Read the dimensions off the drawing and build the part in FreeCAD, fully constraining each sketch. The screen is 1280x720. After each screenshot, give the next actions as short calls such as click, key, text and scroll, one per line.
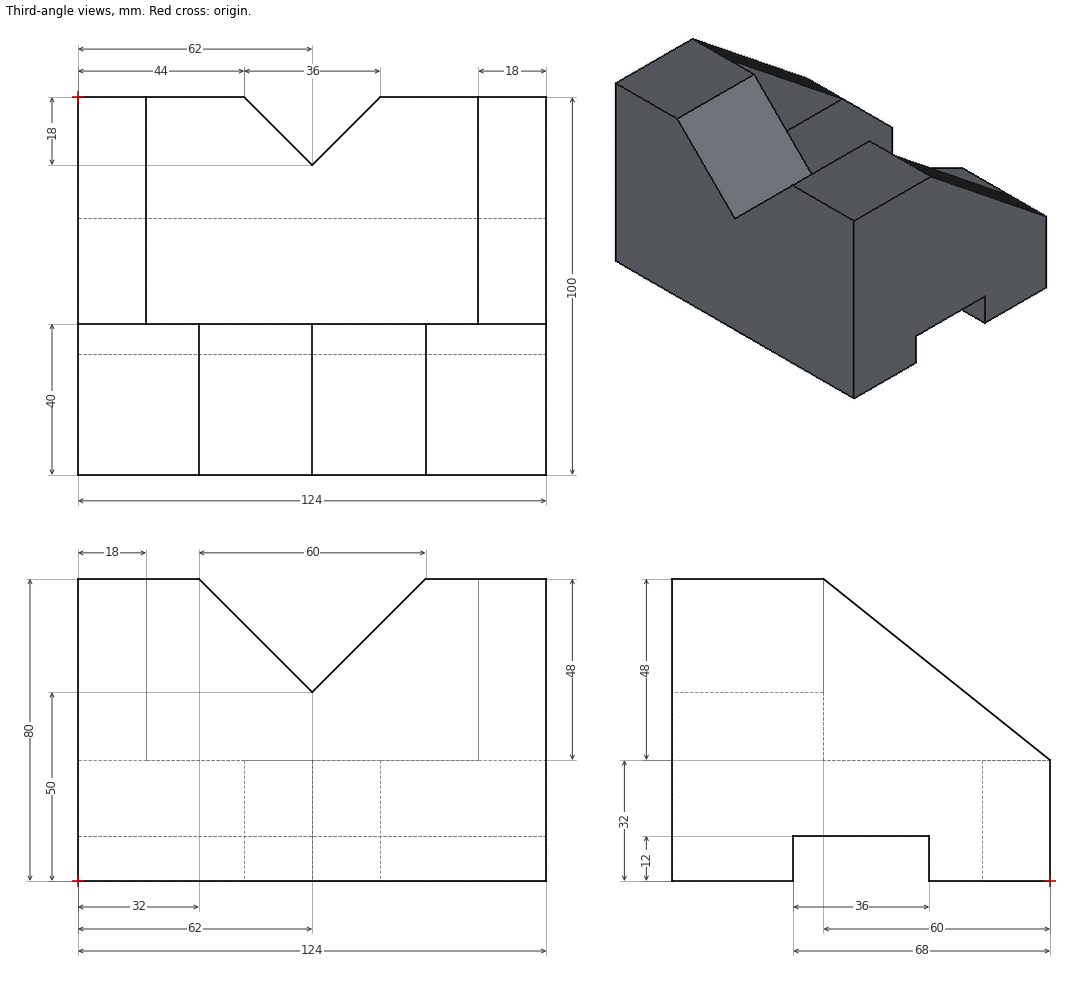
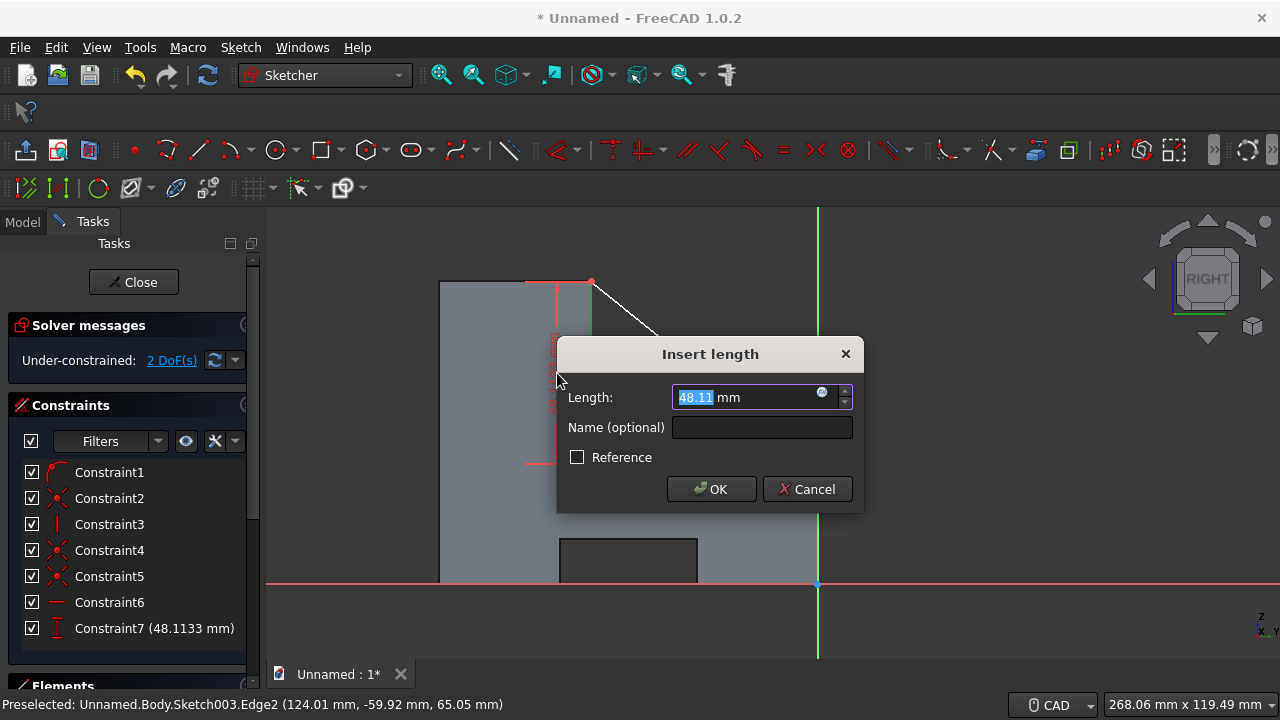
text(48)
key(Return)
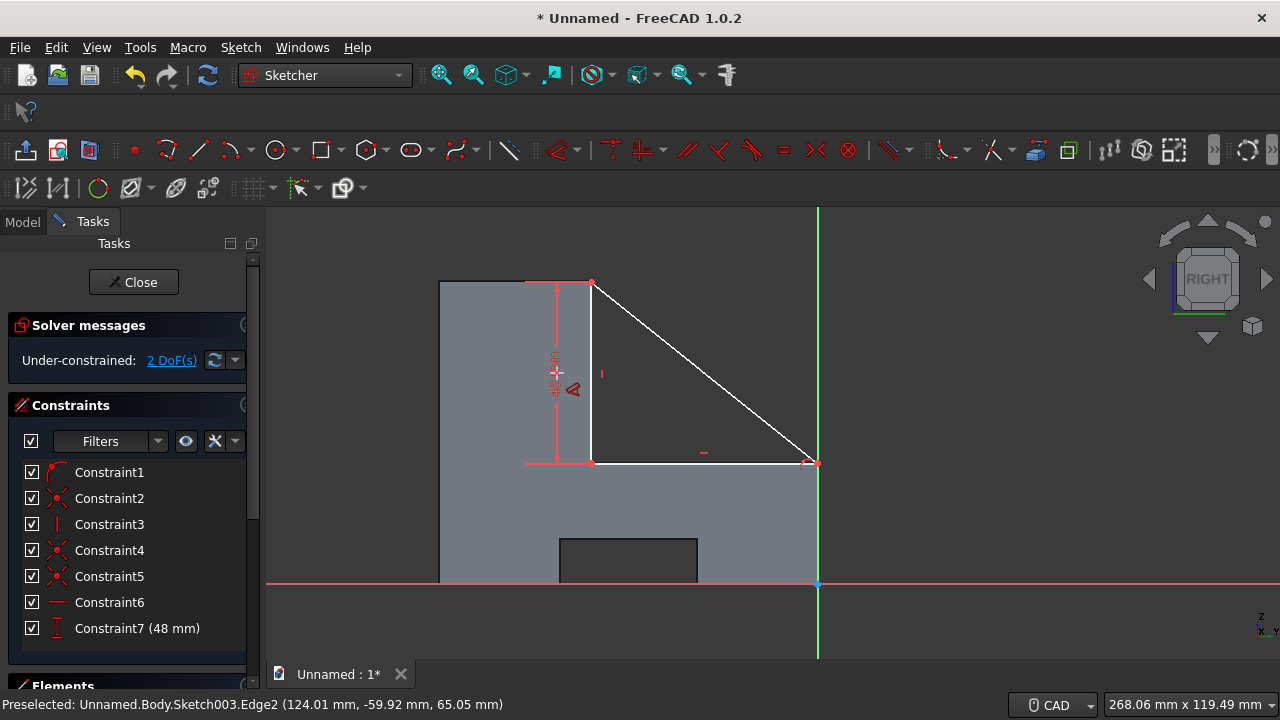
click(659, 464)
click(704, 498)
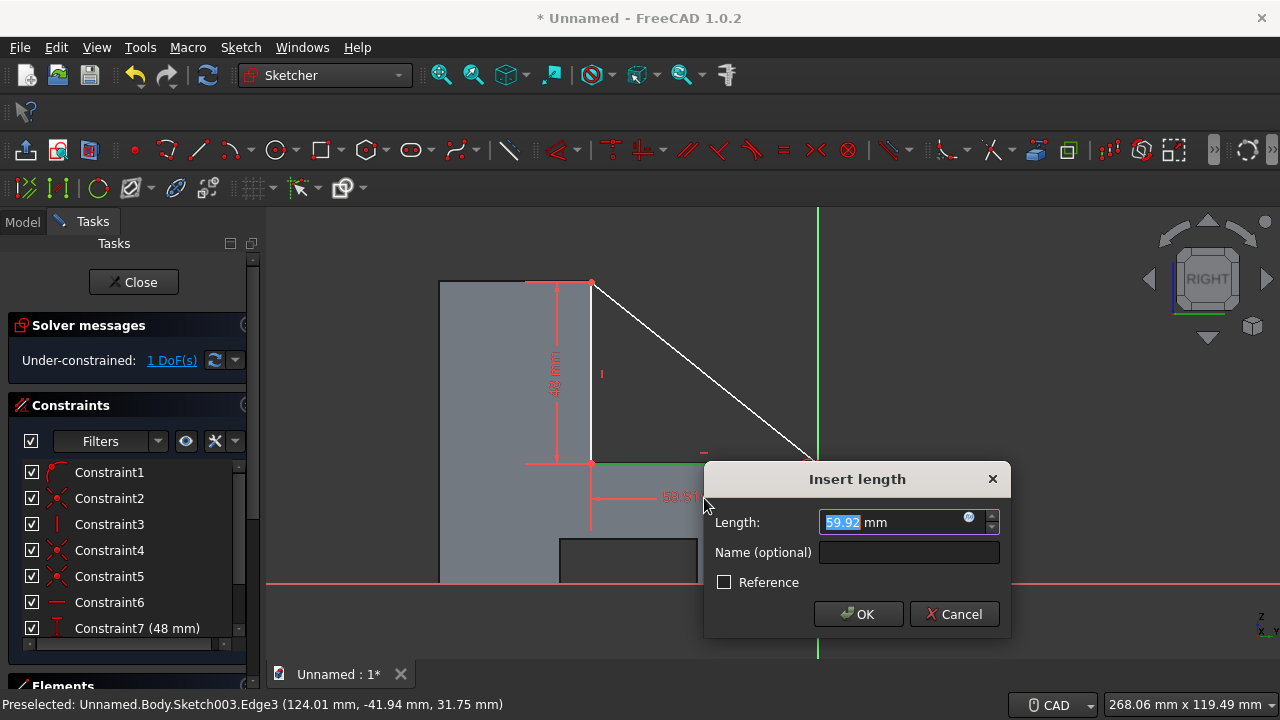
text(60)
key(Return)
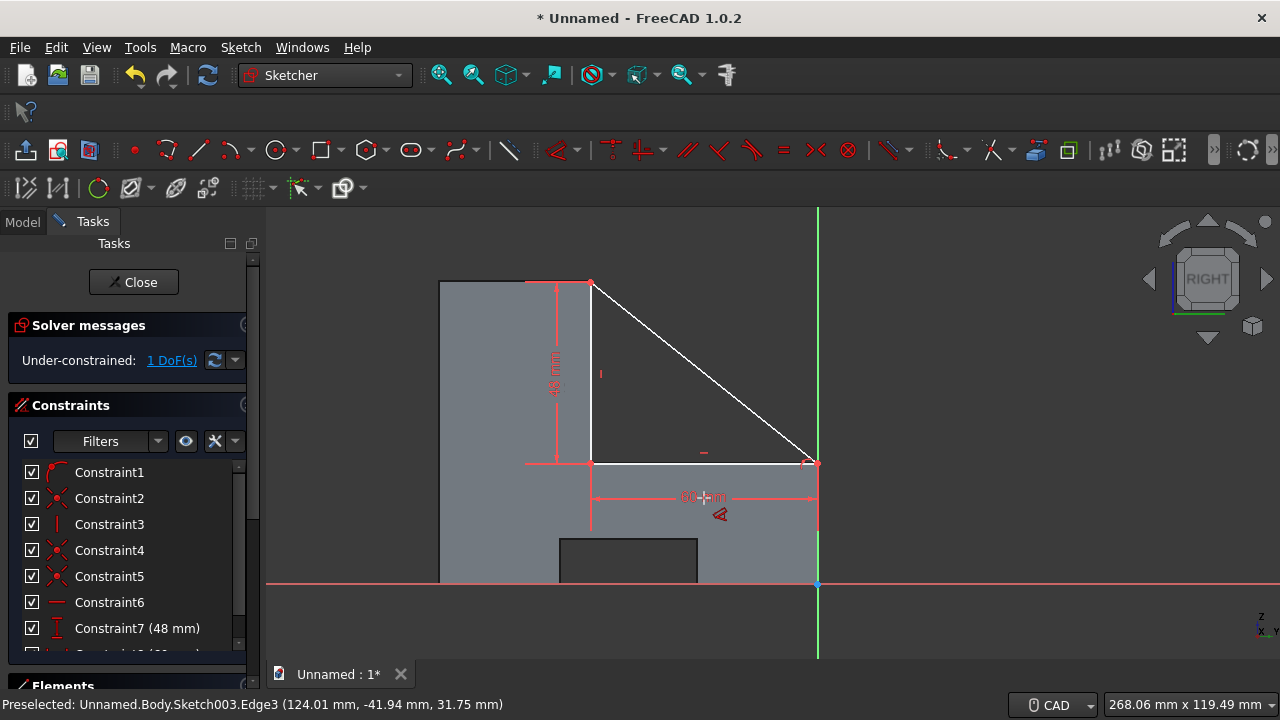
click(818, 464)
click(852, 524)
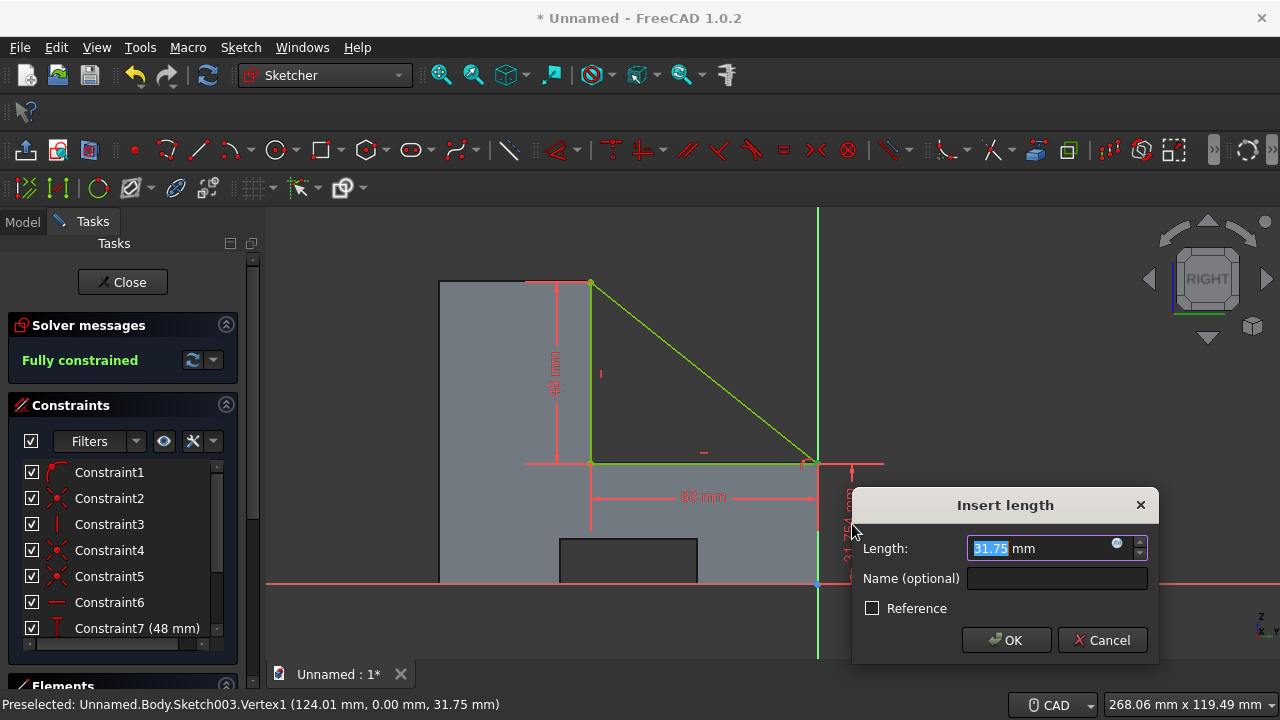
text(32)
key(Return)
key(Escape)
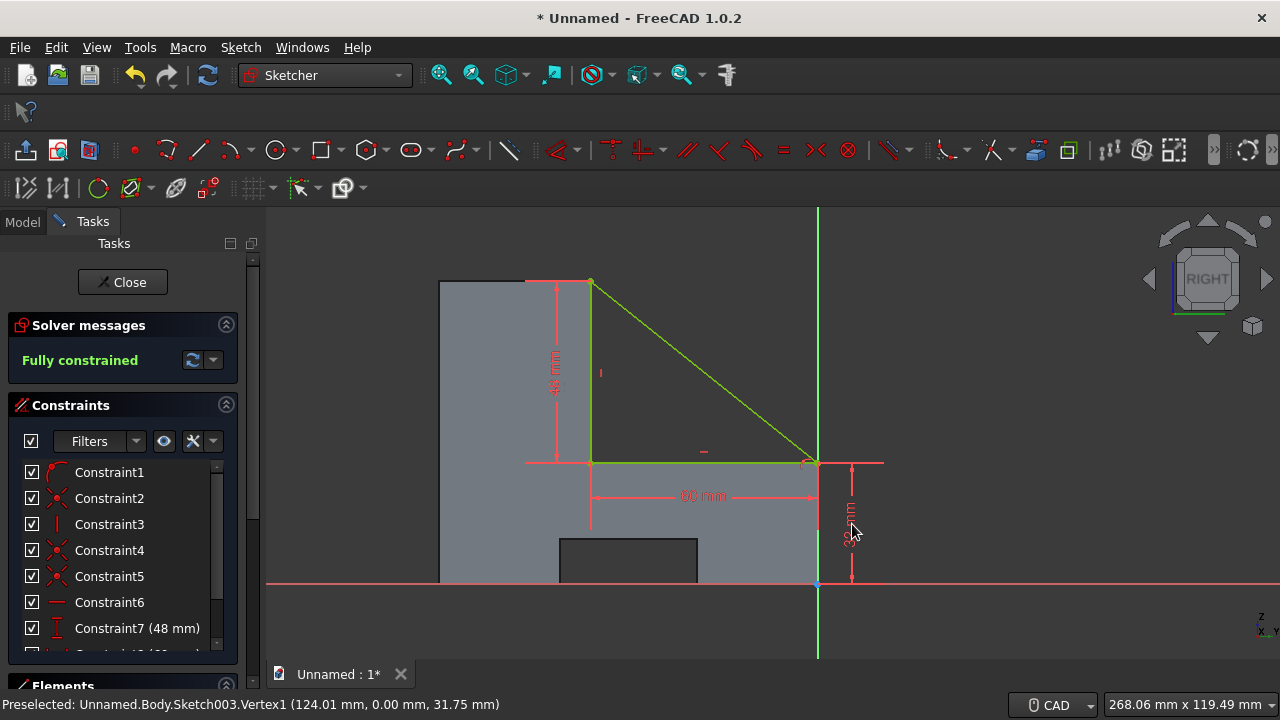
click(123, 282)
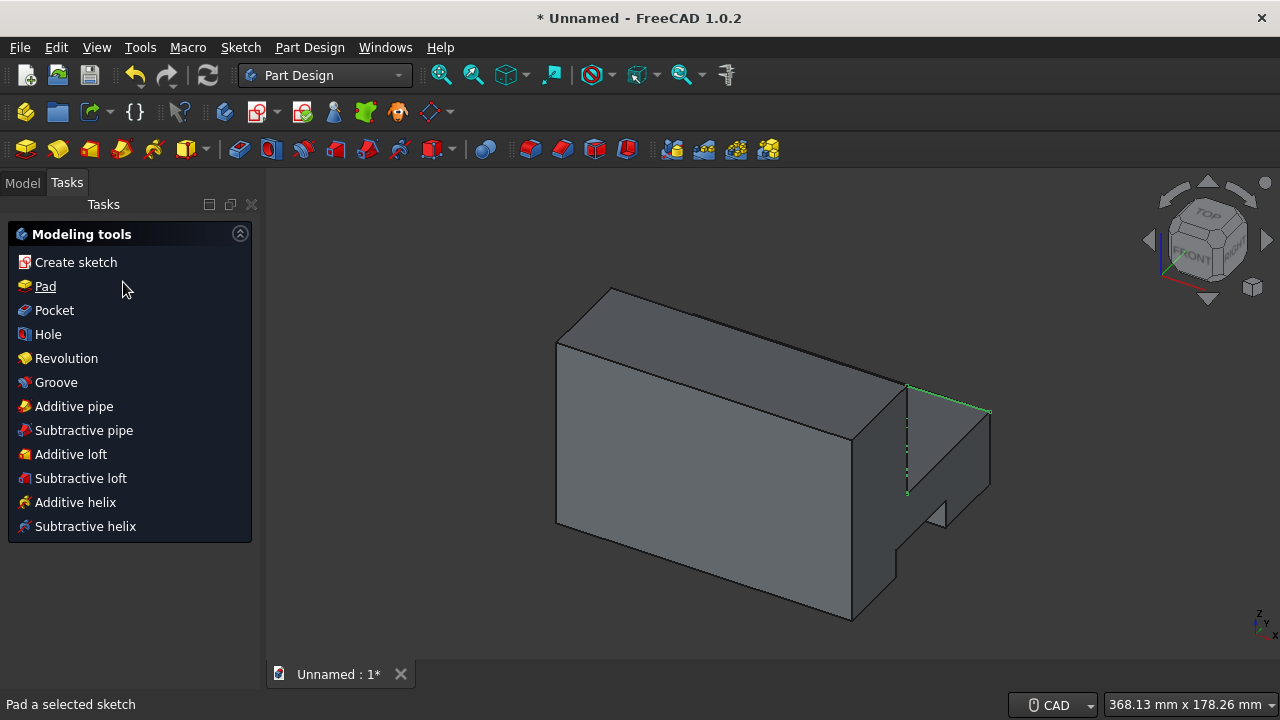
click(26, 150)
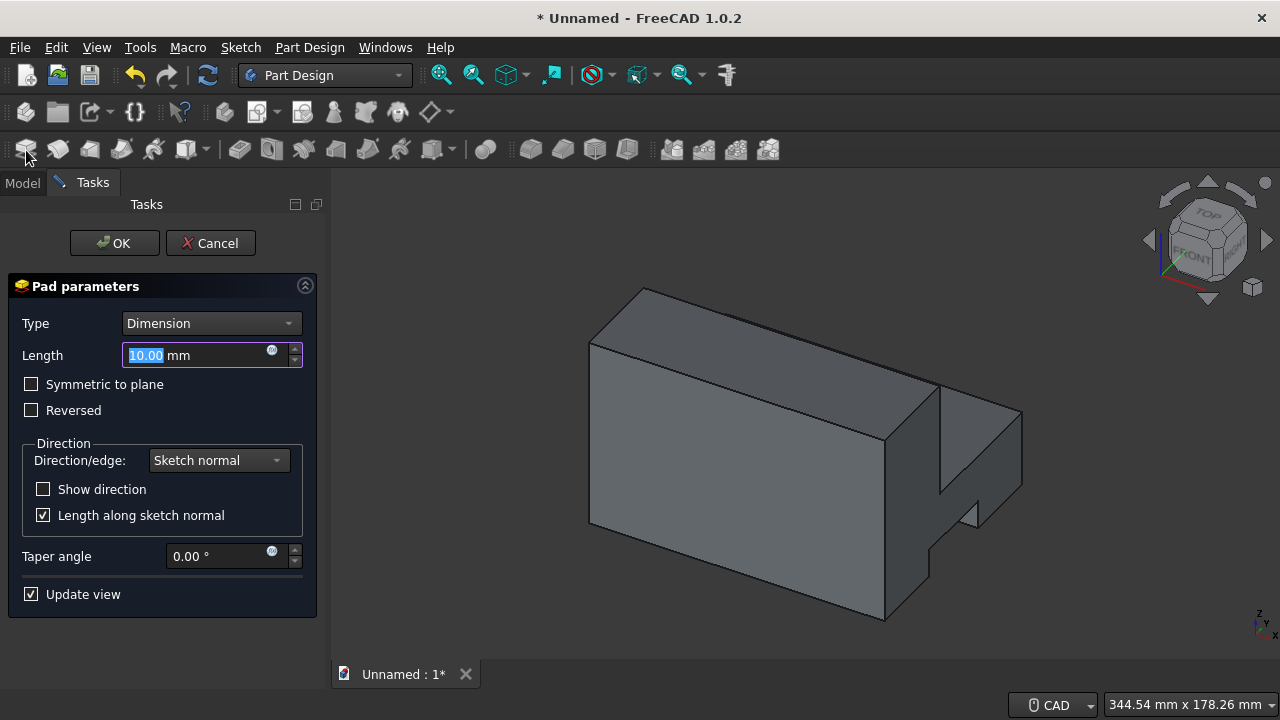
text(18)
key(Tab)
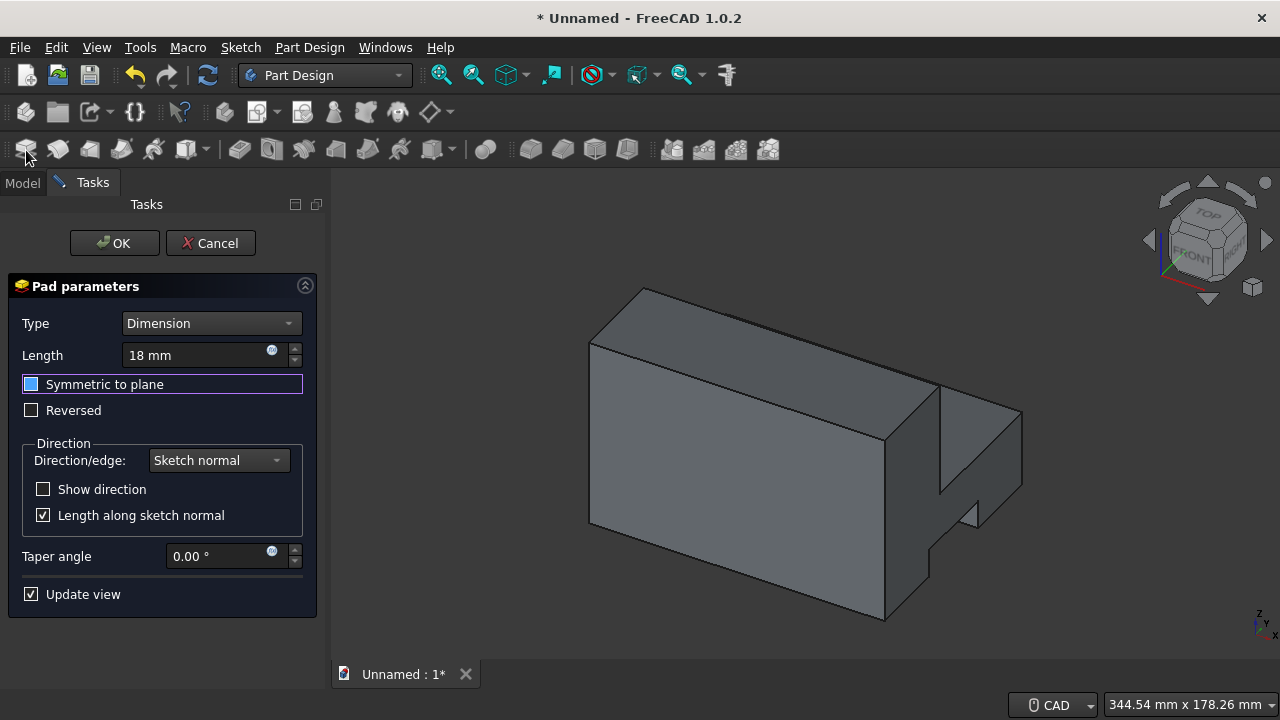
click(30, 410)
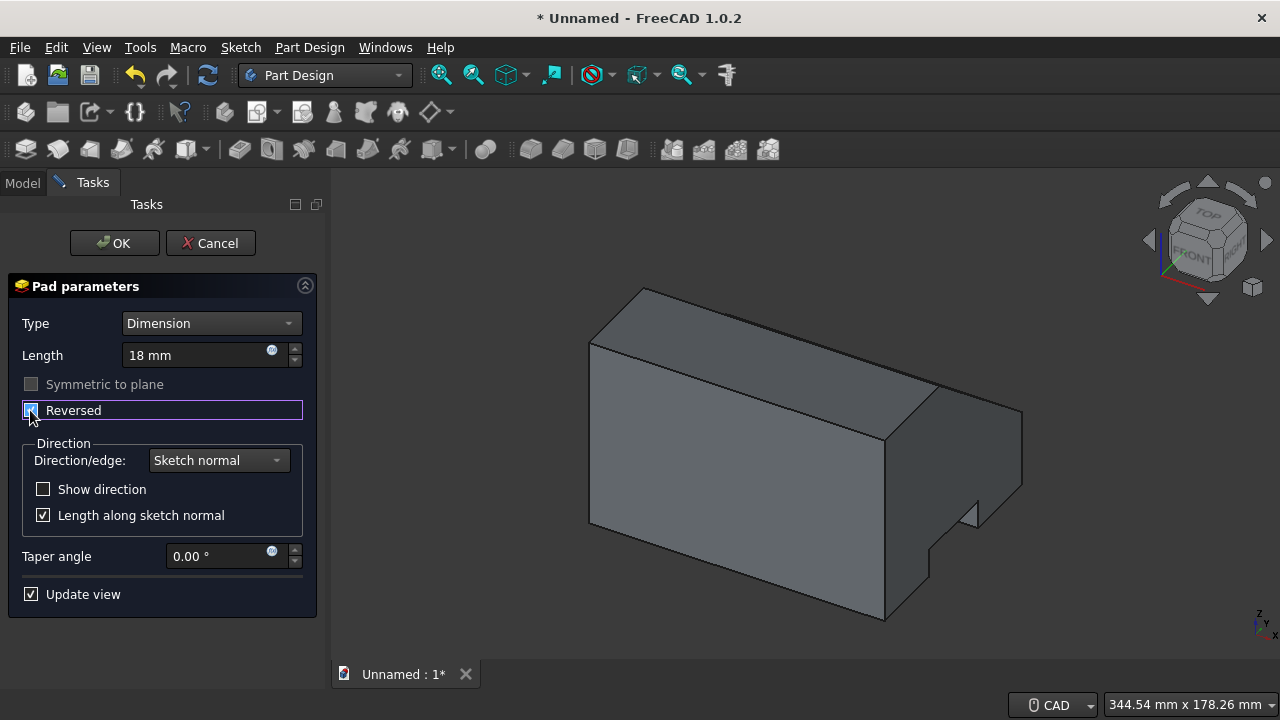
click(115, 243)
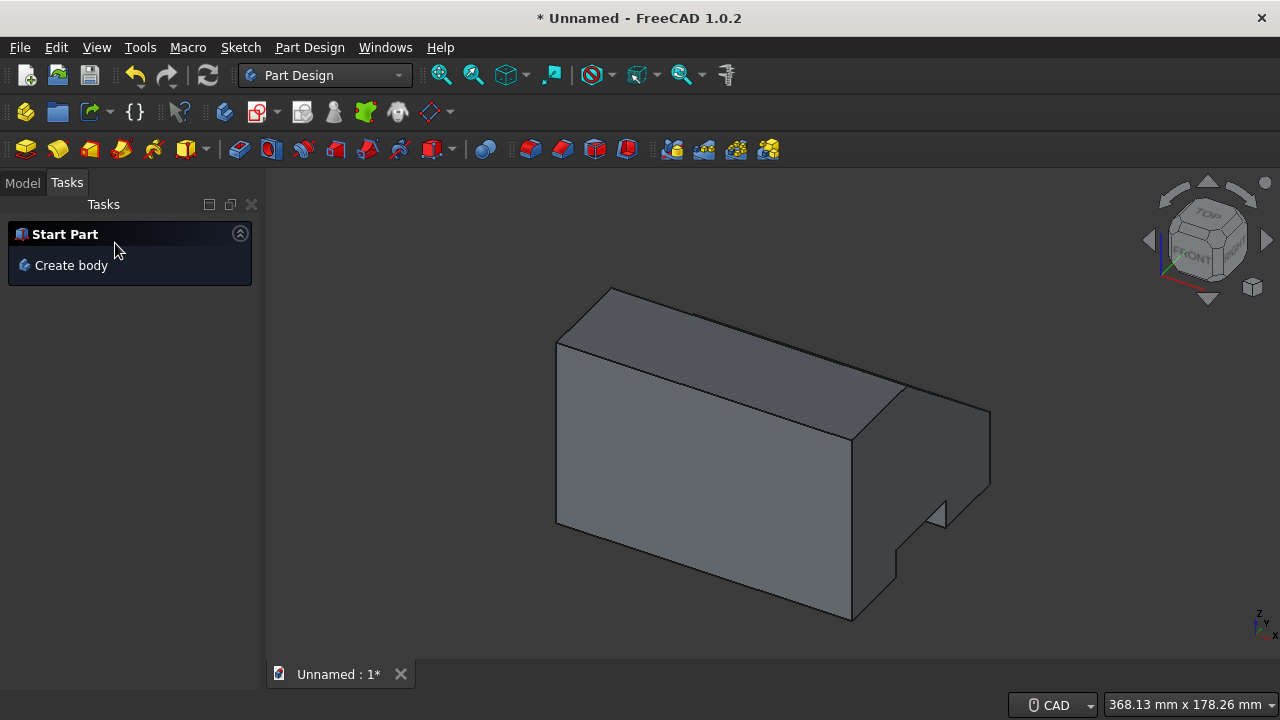
key(6)